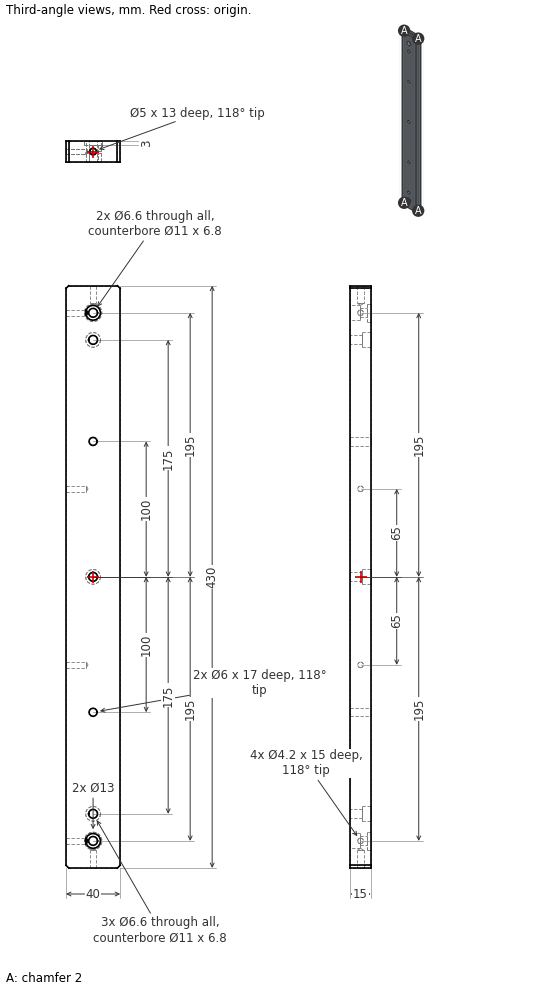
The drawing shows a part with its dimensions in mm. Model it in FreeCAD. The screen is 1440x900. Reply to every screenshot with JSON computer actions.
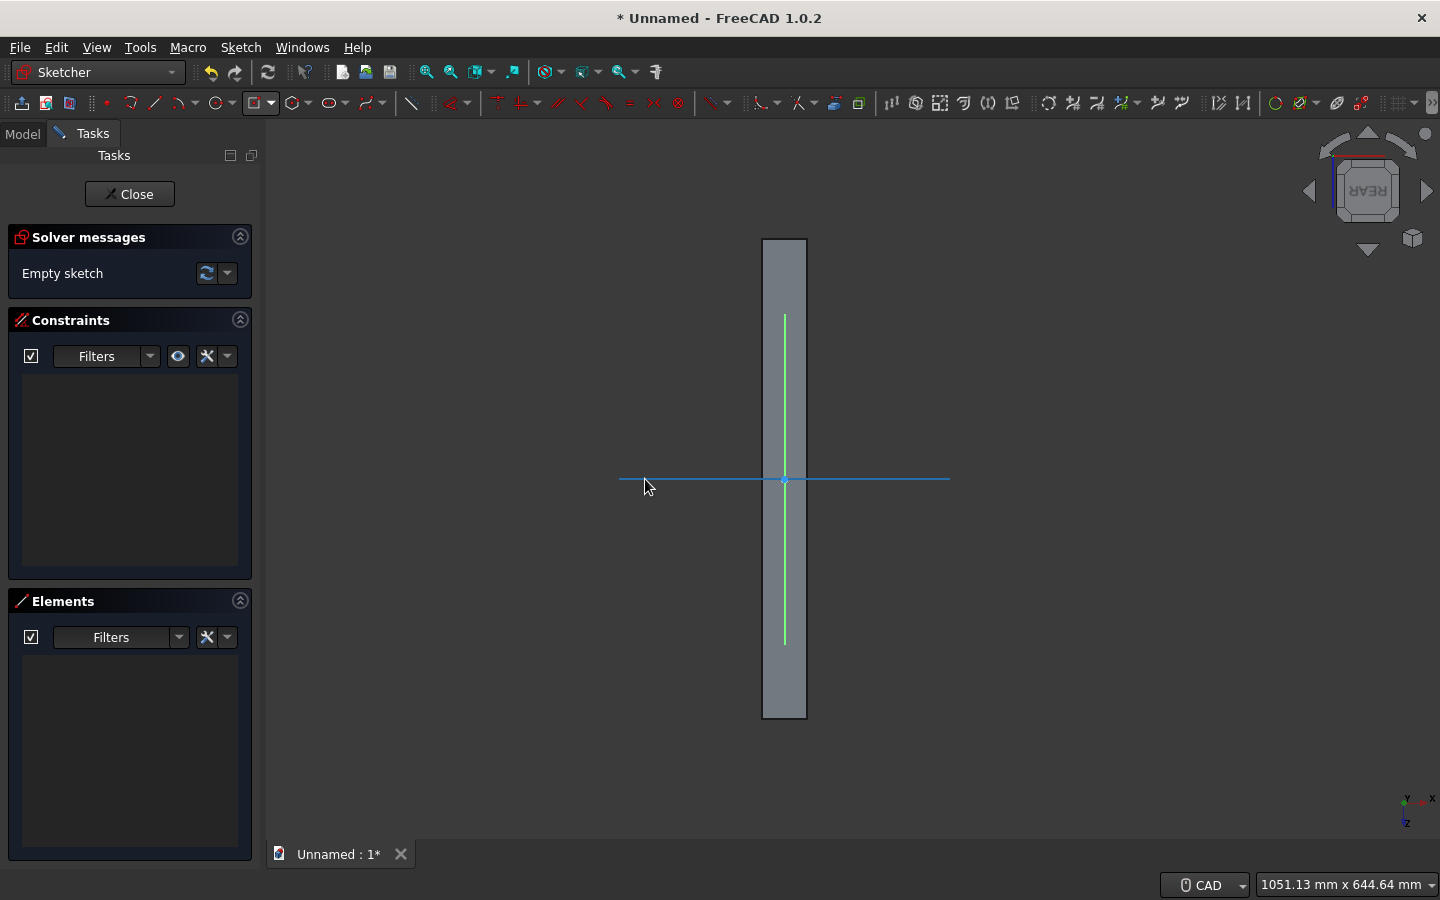
{"action": "left_click", "coordinate": [216, 104]}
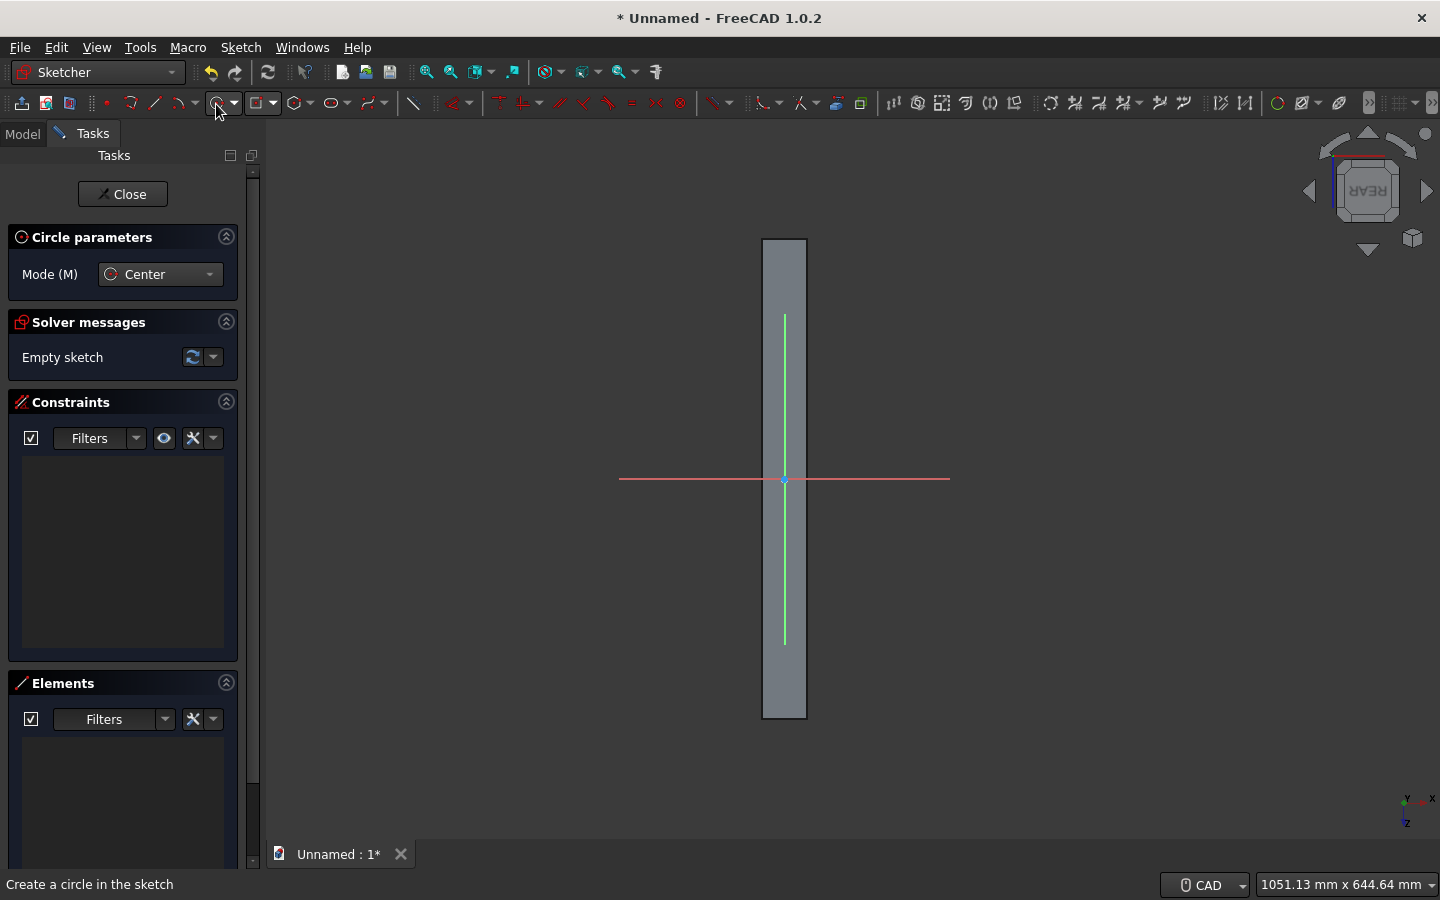
{"action": "scroll", "coordinate": [785, 261], "scroll_direction": "up", "scroll_amount": 6}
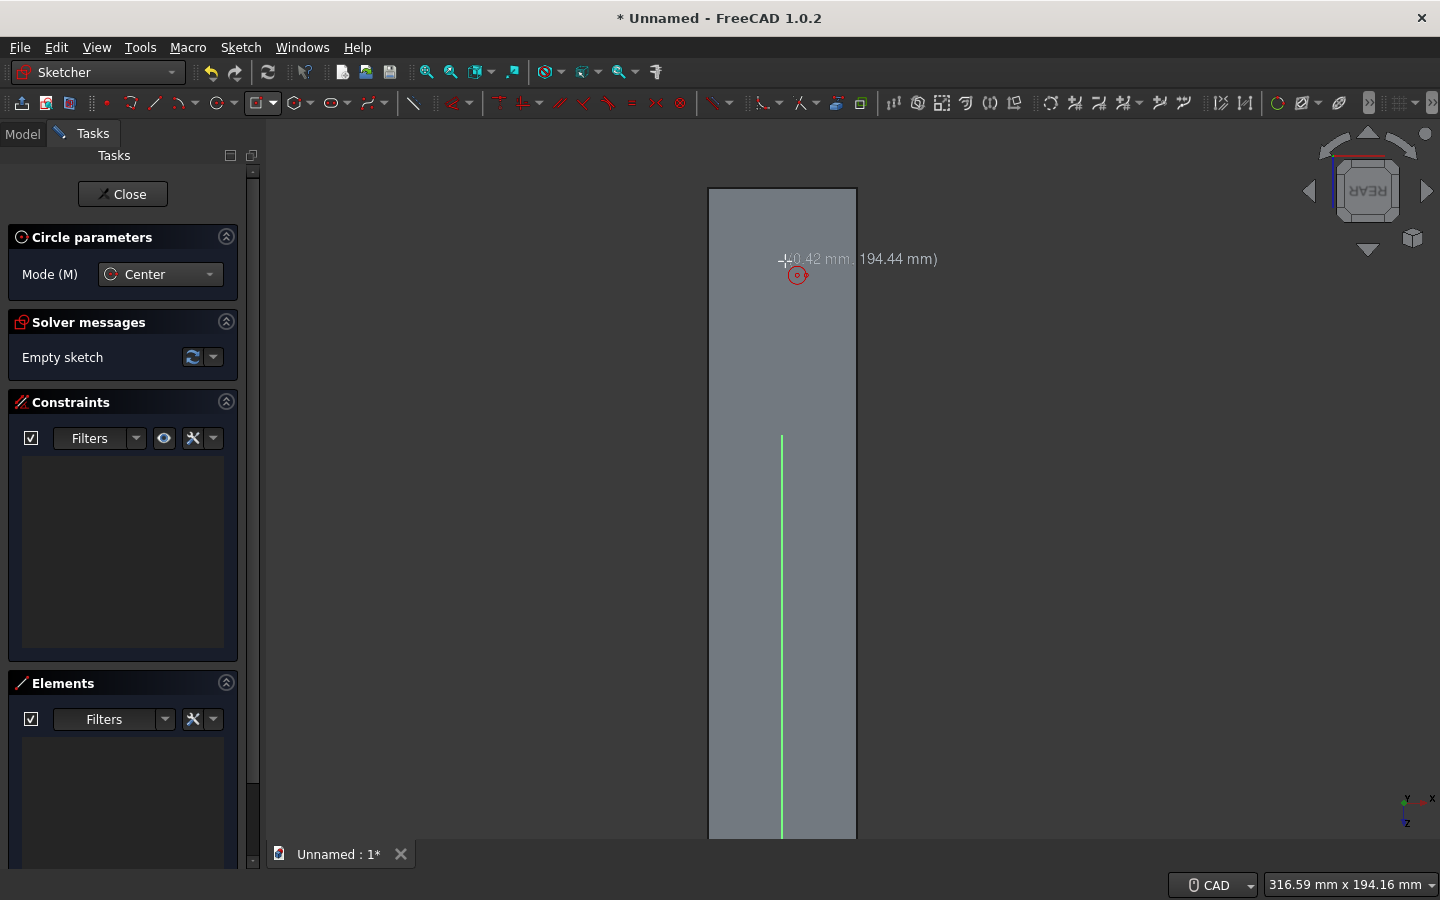
{"action": "left_click", "coordinate": [782, 262]}
{"action": "left_click", "coordinate": [799, 245]}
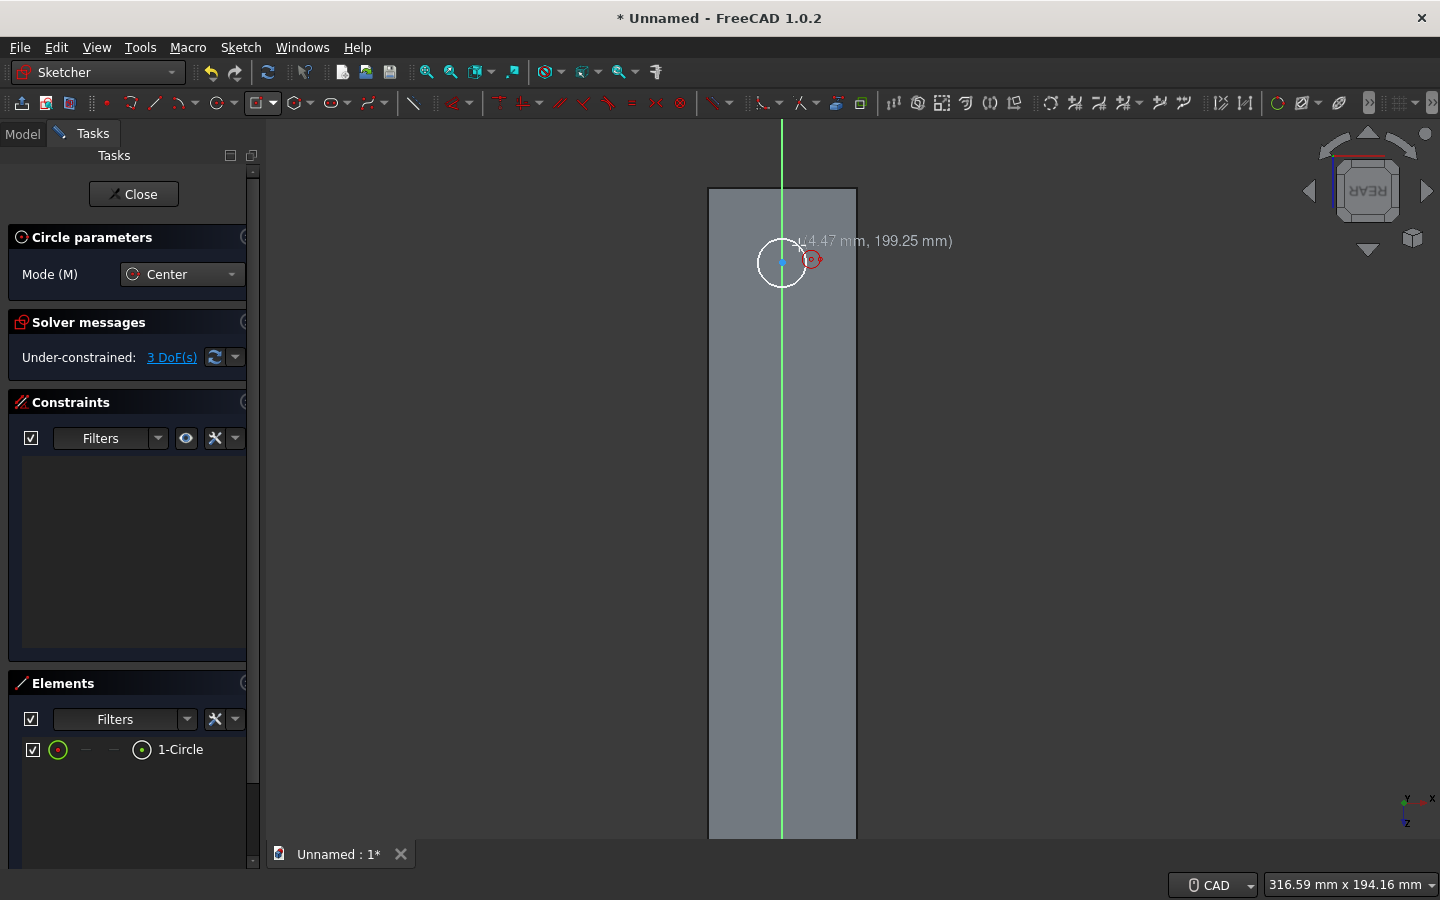
{"action": "scroll", "coordinate": [785, 261], "scroll_direction": "down", "scroll_amount": 6}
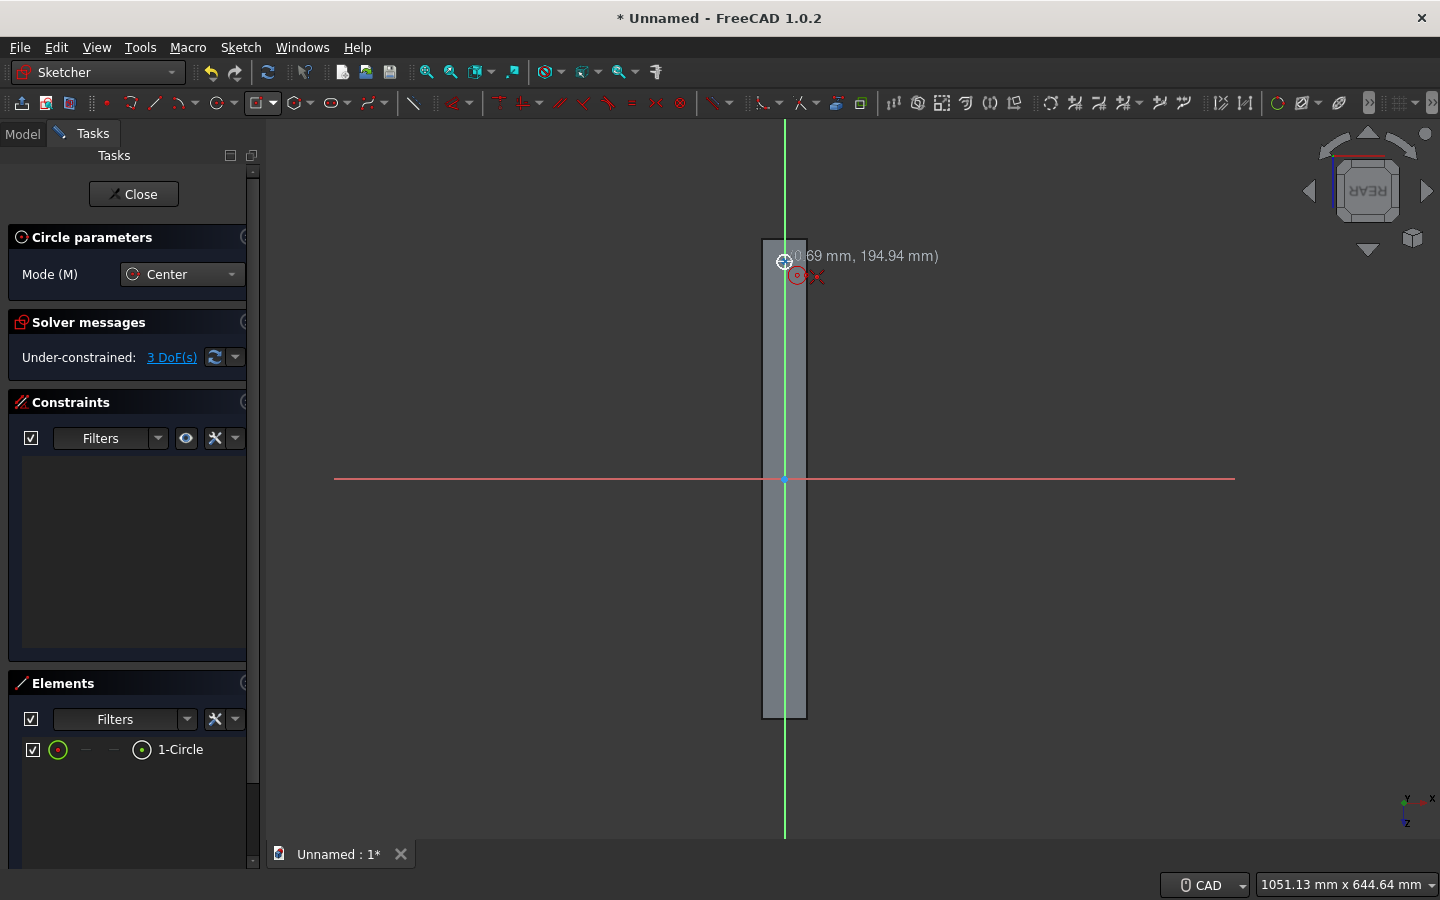
{"action": "scroll", "coordinate": [785, 697], "scroll_direction": "up", "scroll_amount": 6}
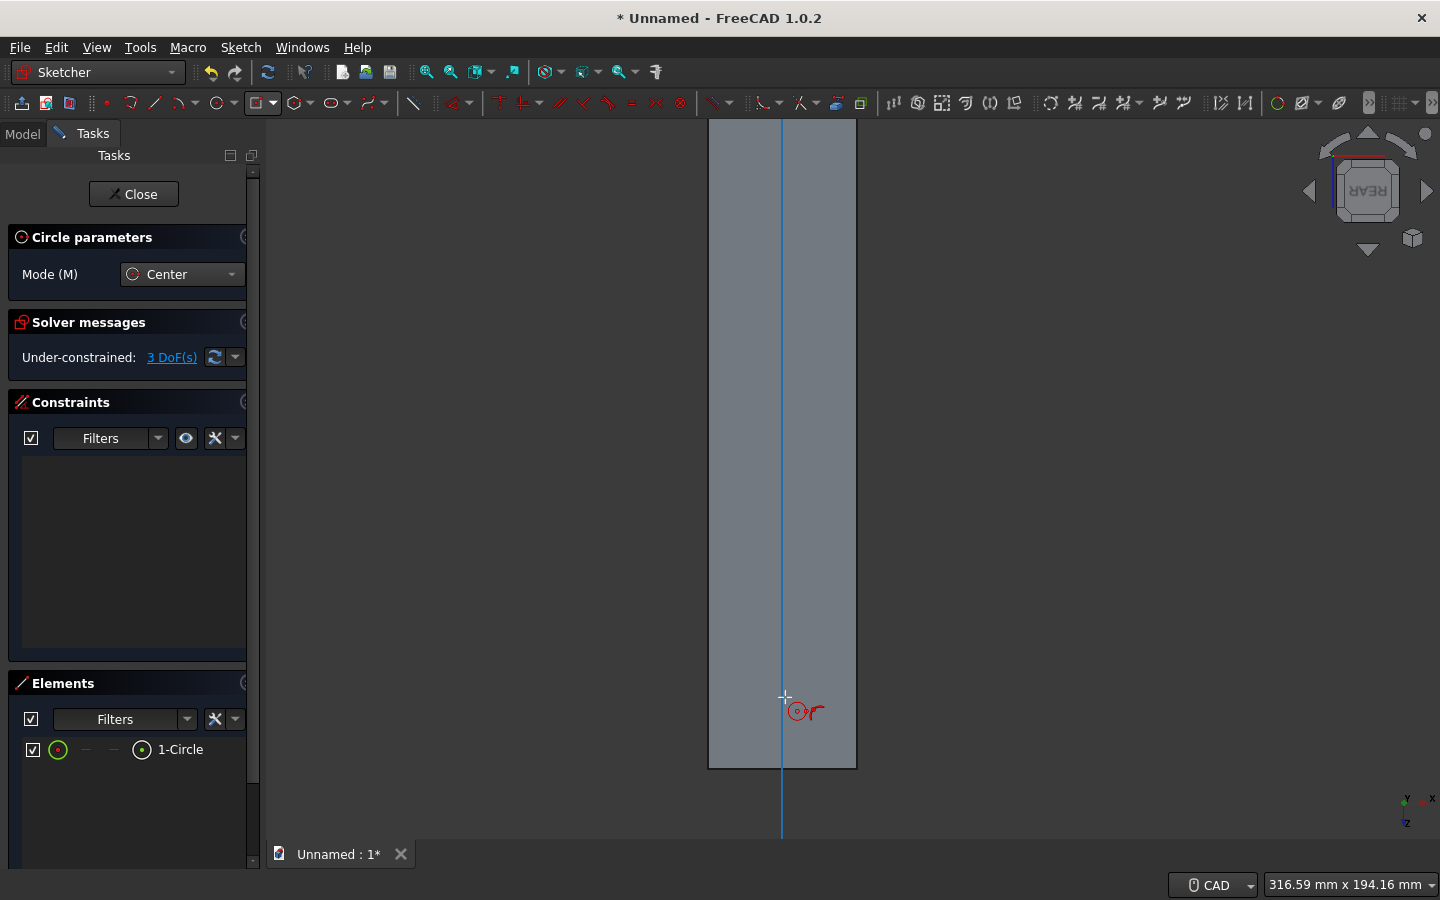
{"action": "left_click", "coordinate": [782, 695]}
{"action": "left_click", "coordinate": [799, 678]}
{"action": "key", "text": "Escape"}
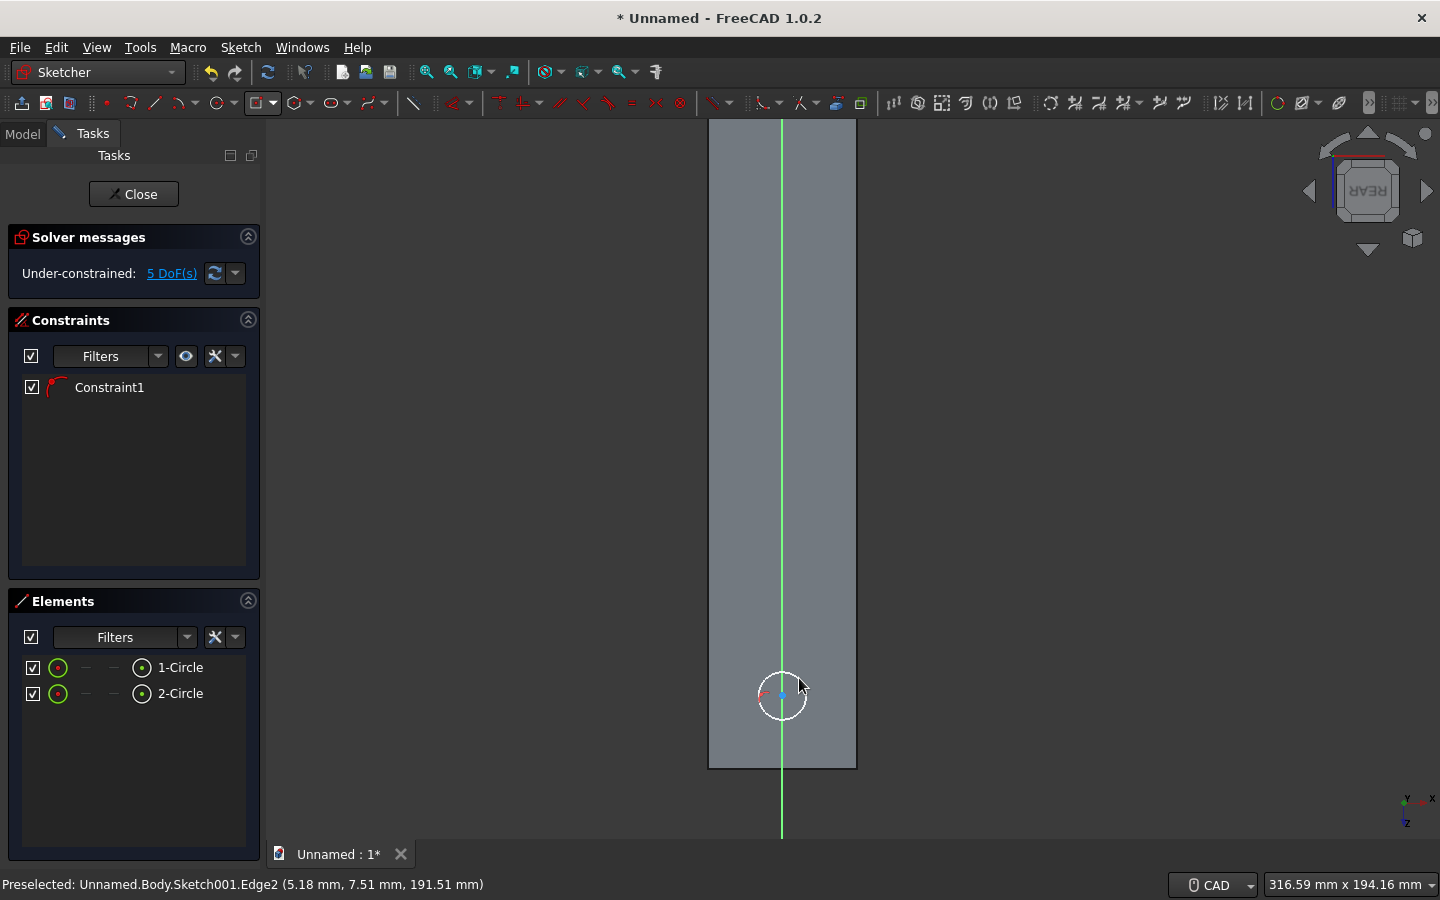
{"action": "scroll", "coordinate": [785, 698], "scroll_direction": "down", "scroll_amount": 6}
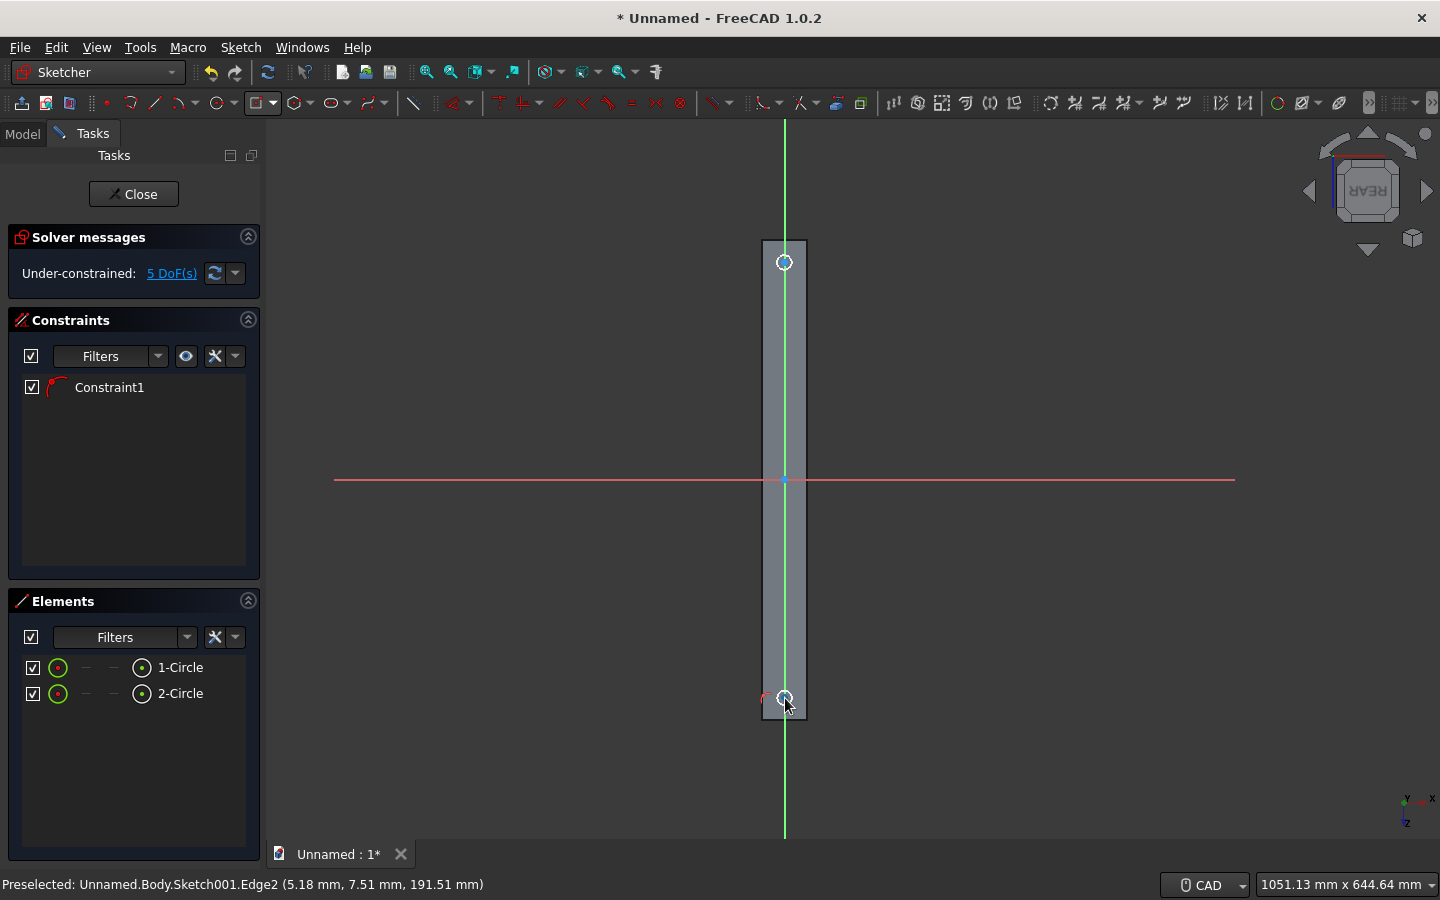
{"action": "scroll", "coordinate": [790, 257], "scroll_direction": "up", "scroll_amount": 6}